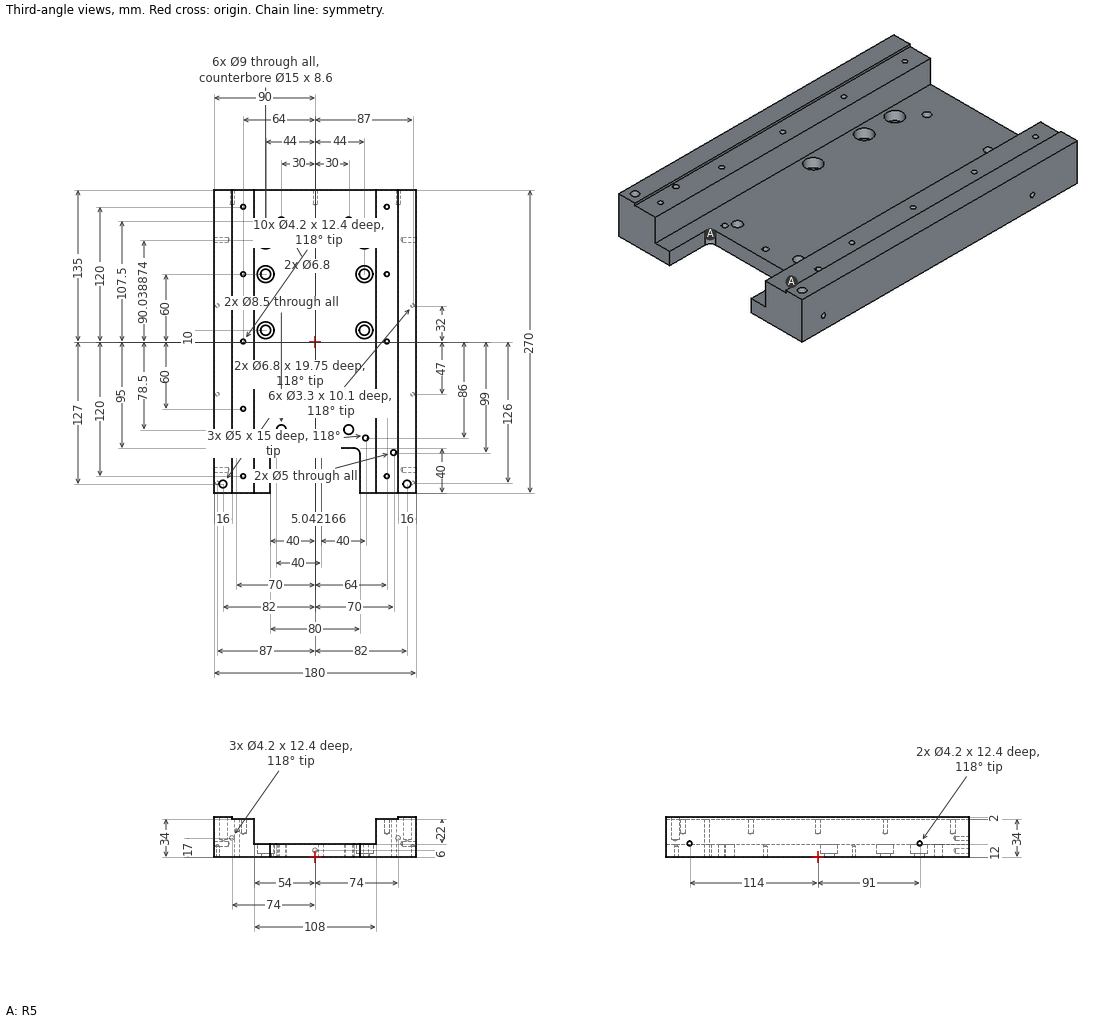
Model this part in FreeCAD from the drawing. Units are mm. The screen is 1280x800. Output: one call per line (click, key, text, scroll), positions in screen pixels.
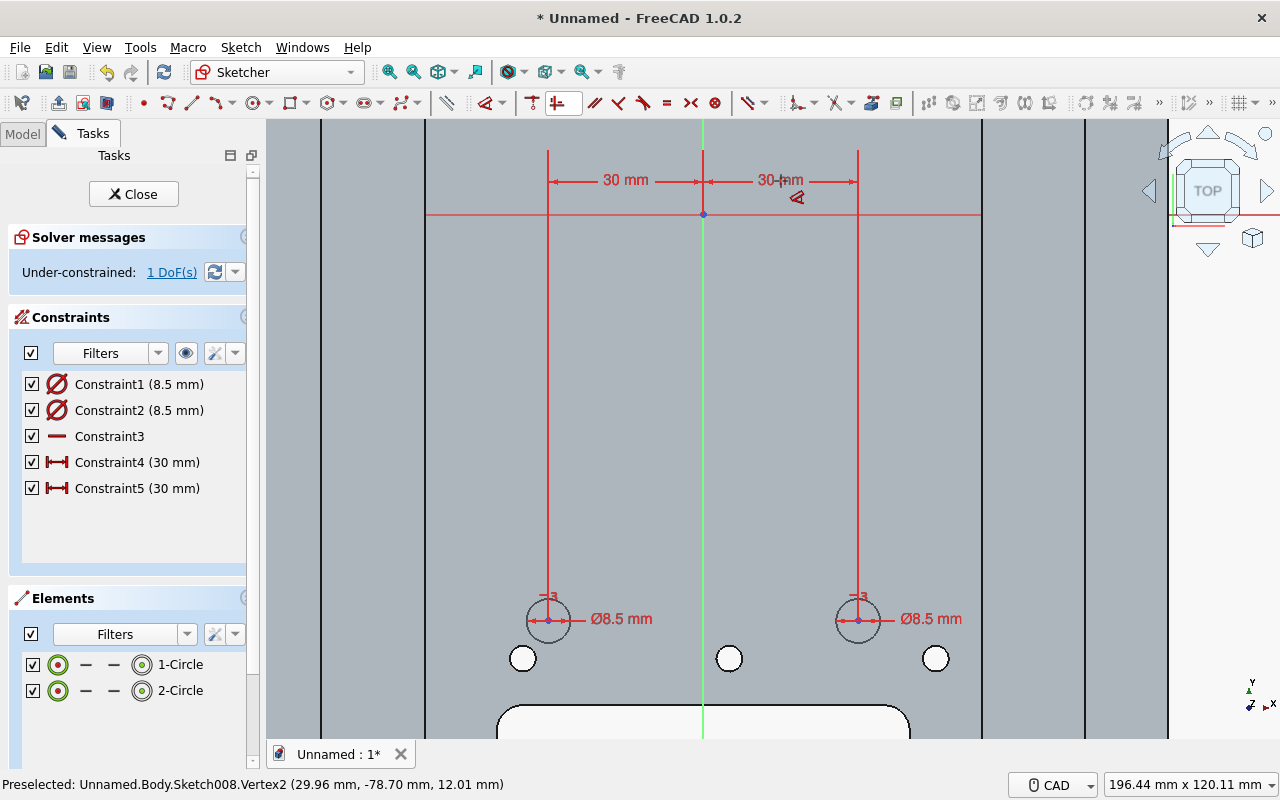
click(548, 621)
click(514, 418)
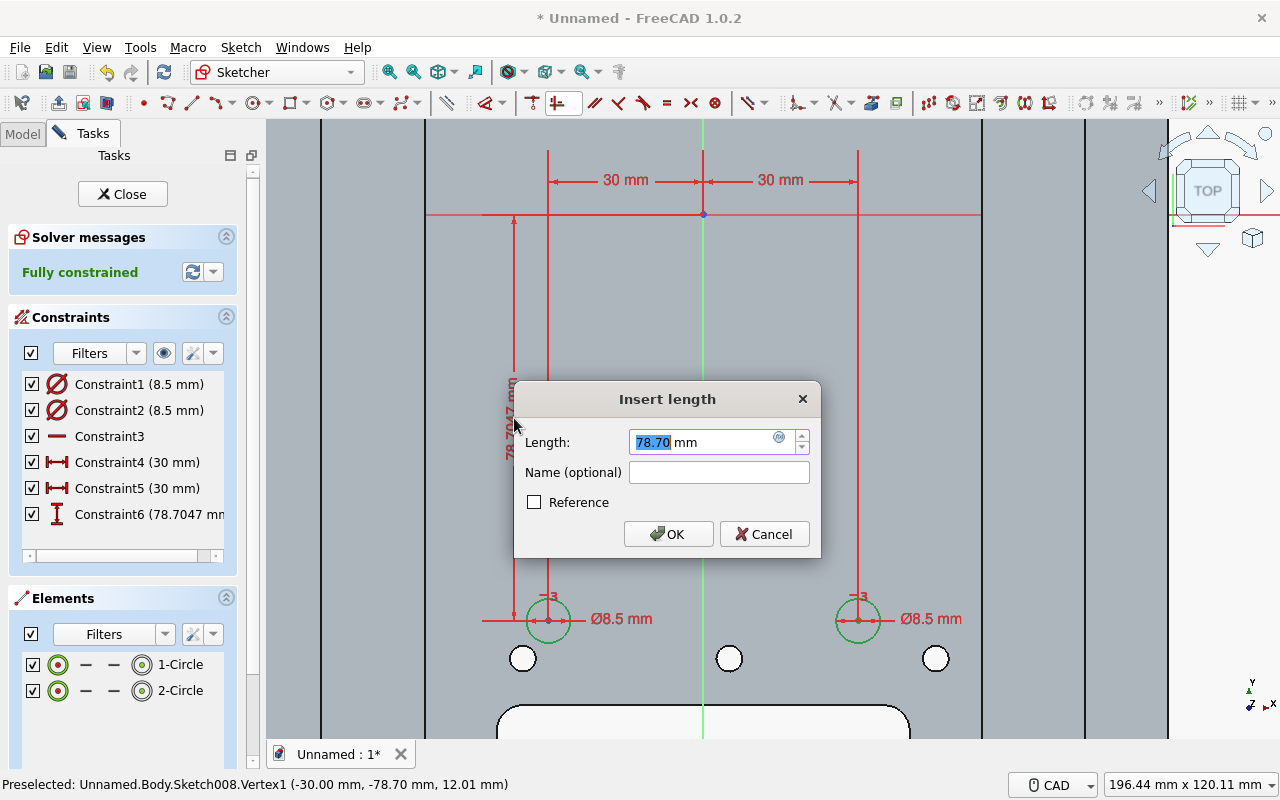
text(78.5)
key(Return)
key(Escape)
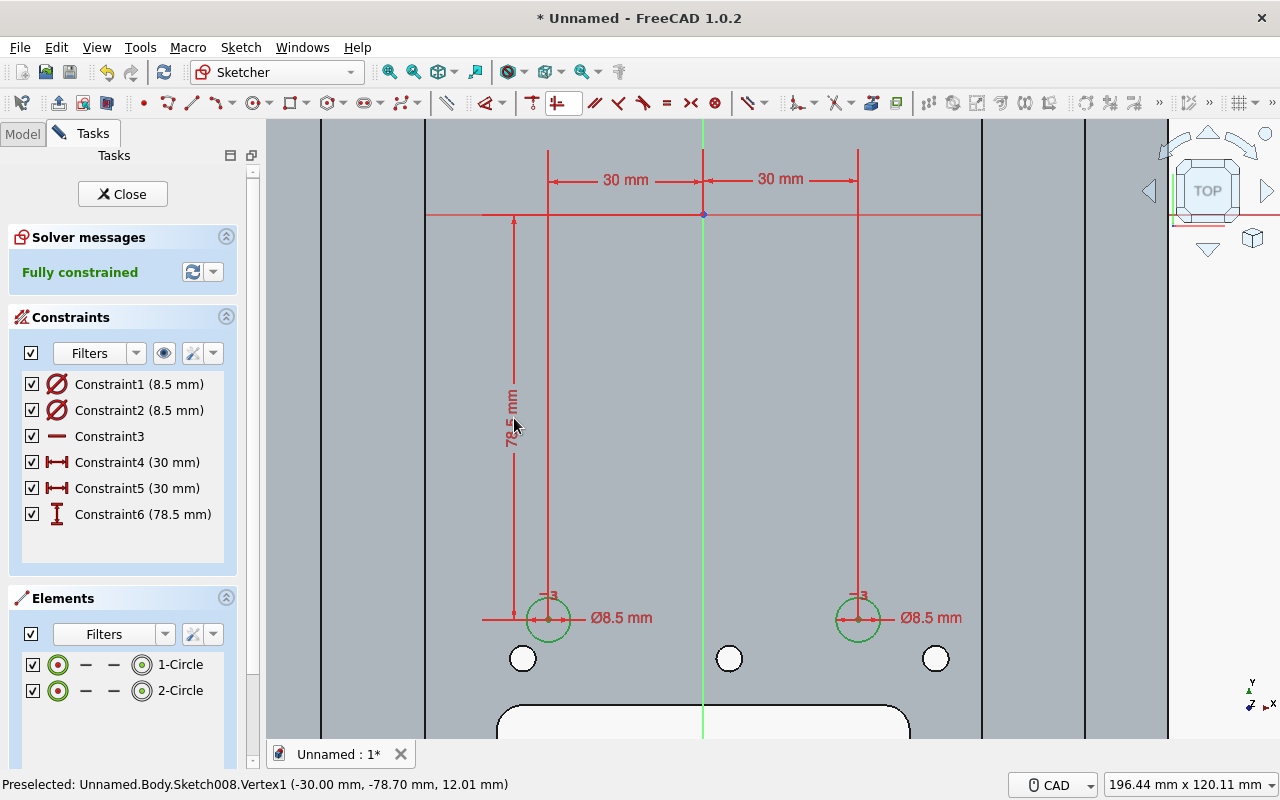
click(123, 194)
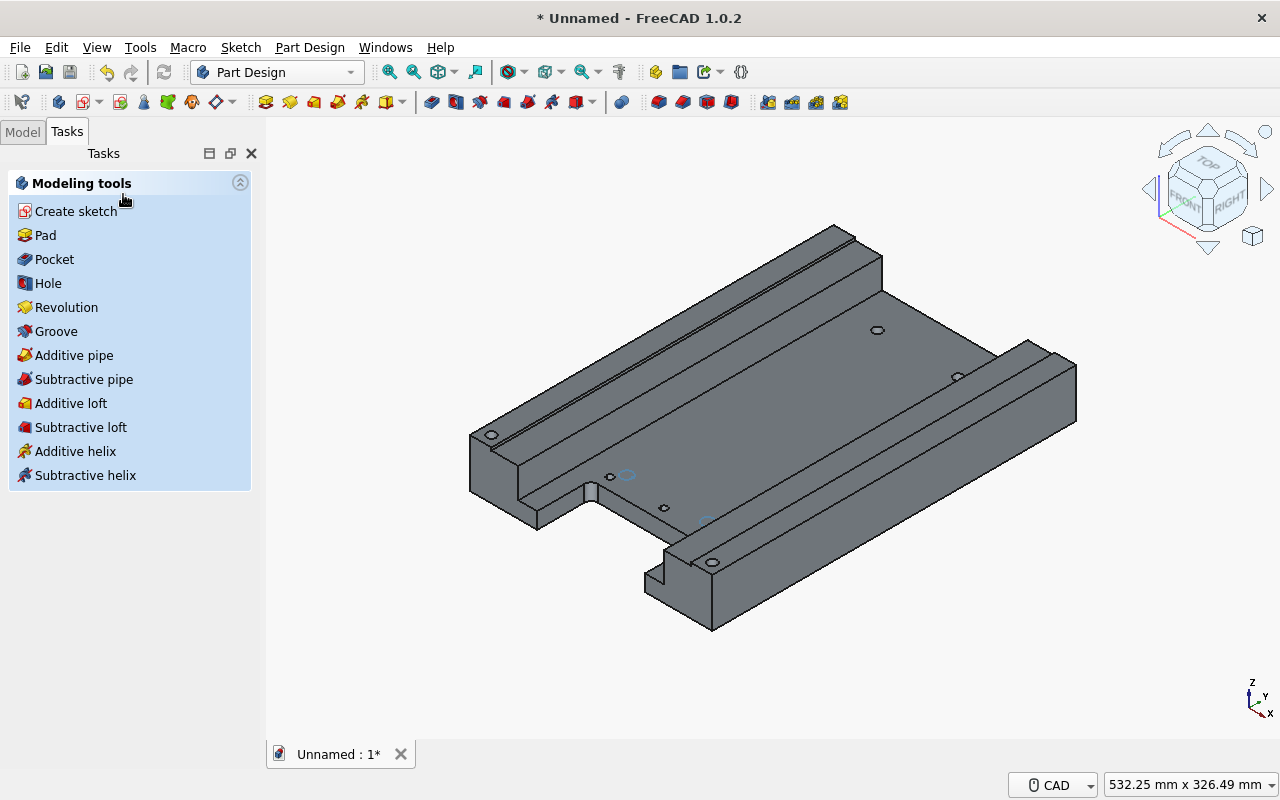
click(456, 102)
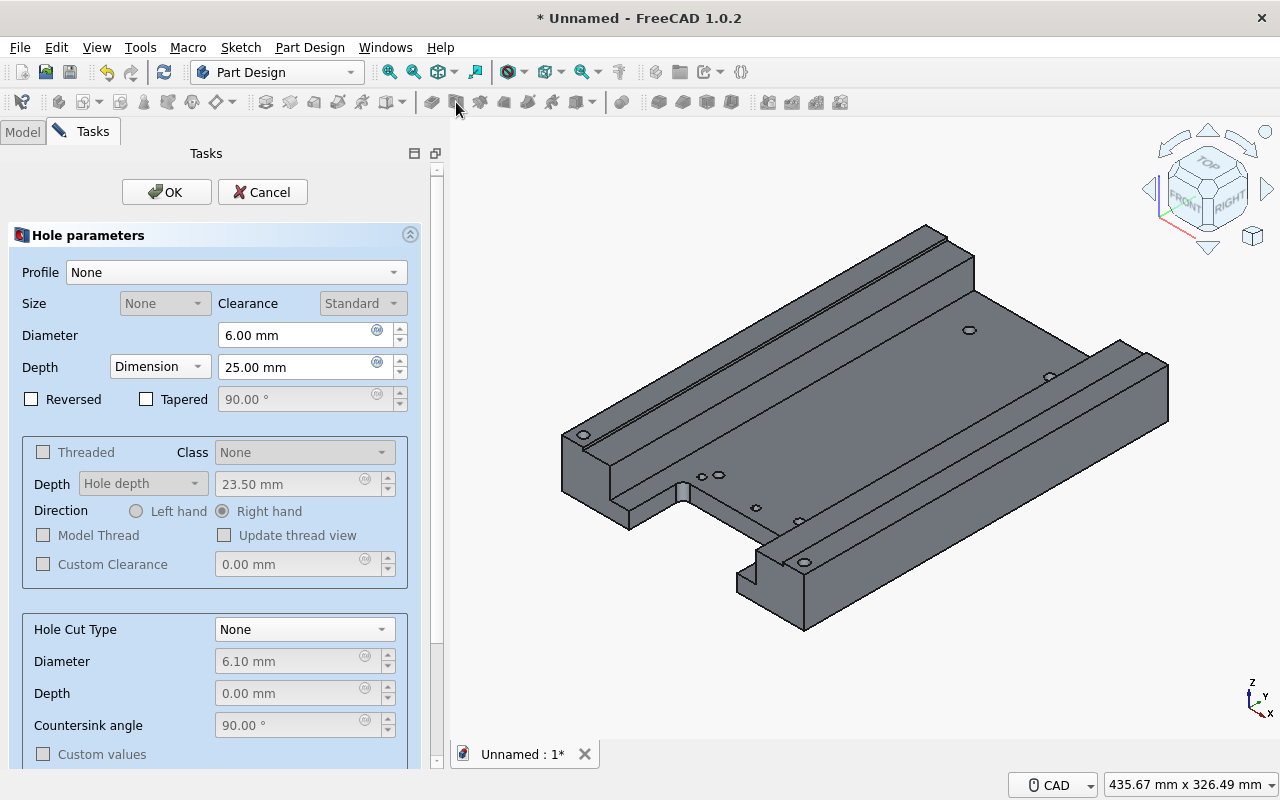
triple_click(305, 335)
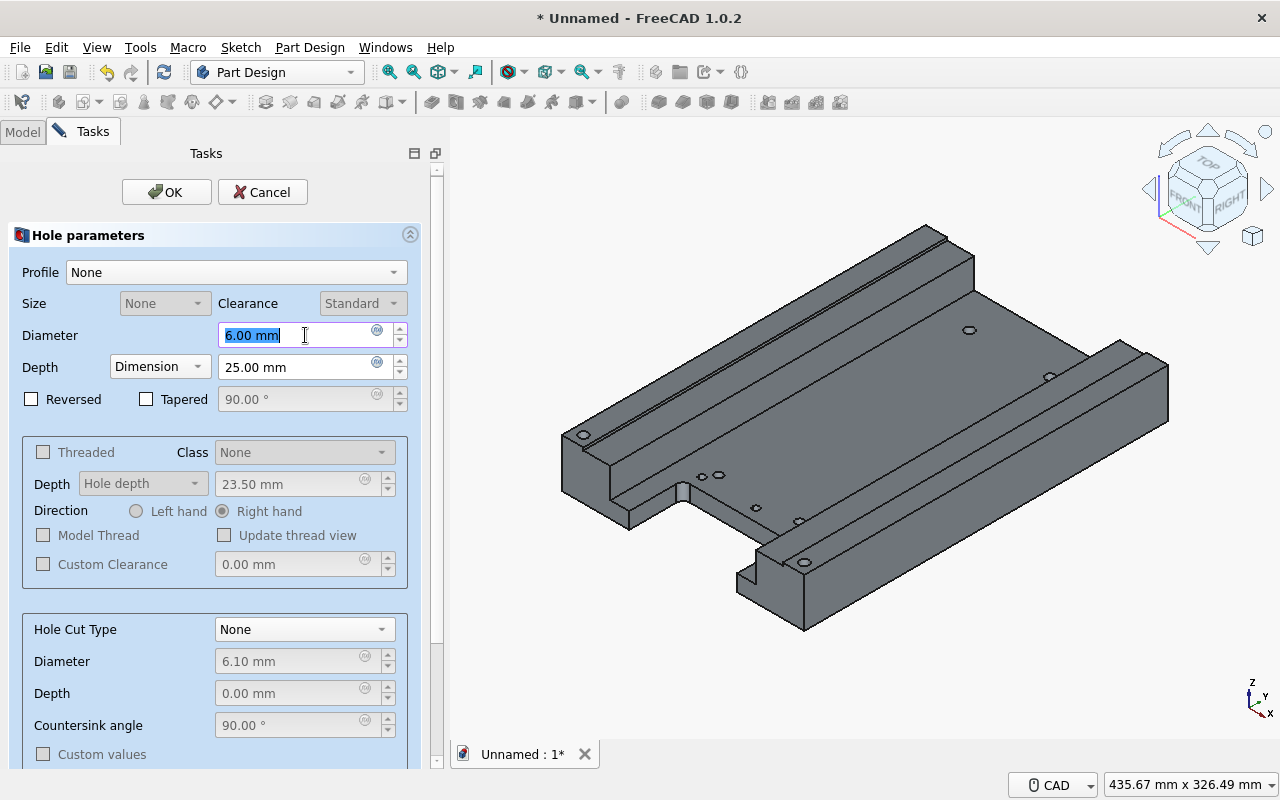
text(8.5)
key(Tab)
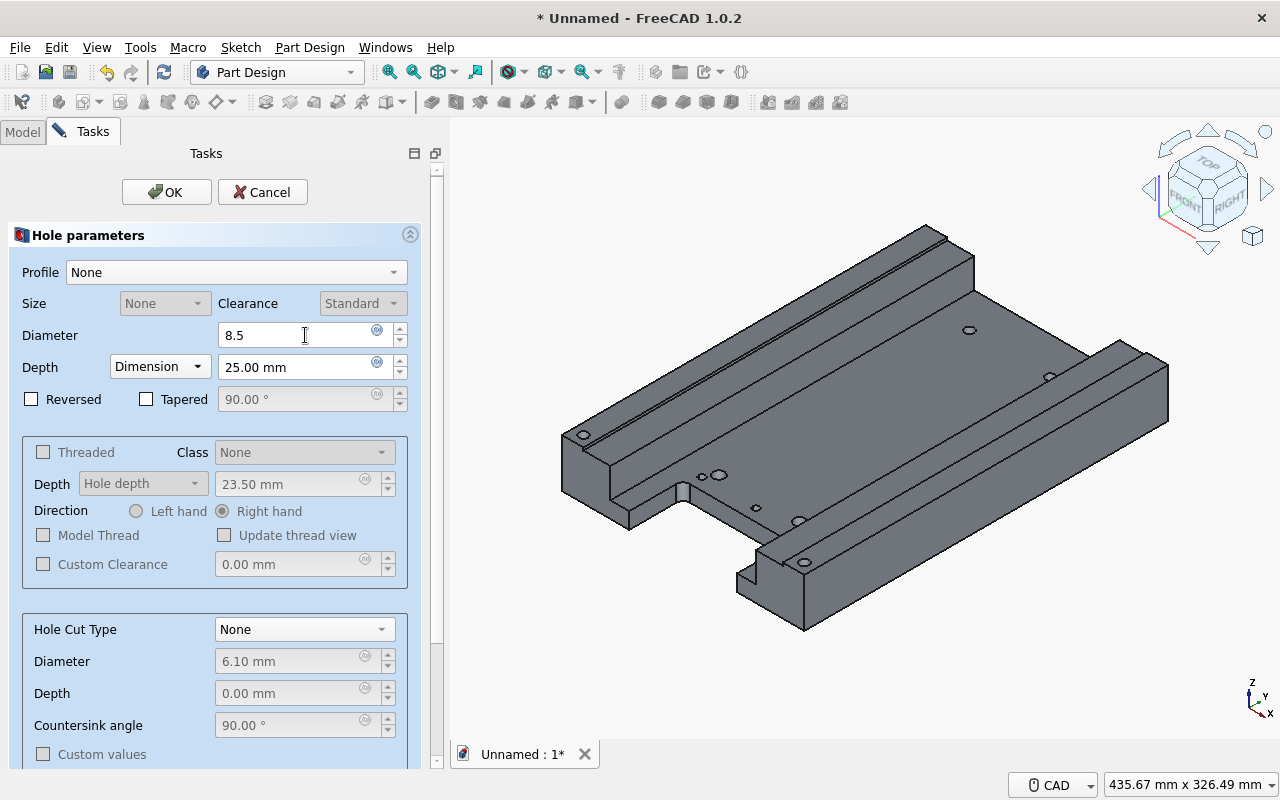
click(161, 366)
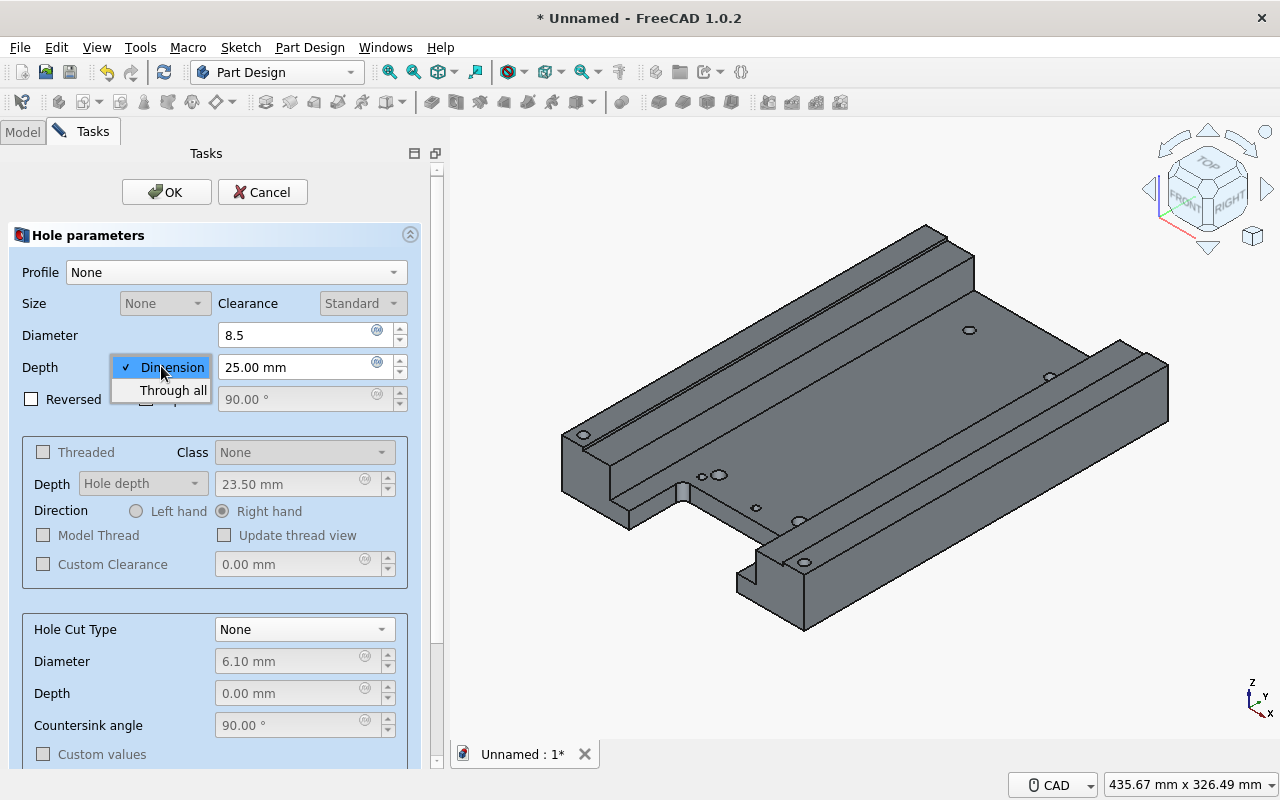
click(160, 390)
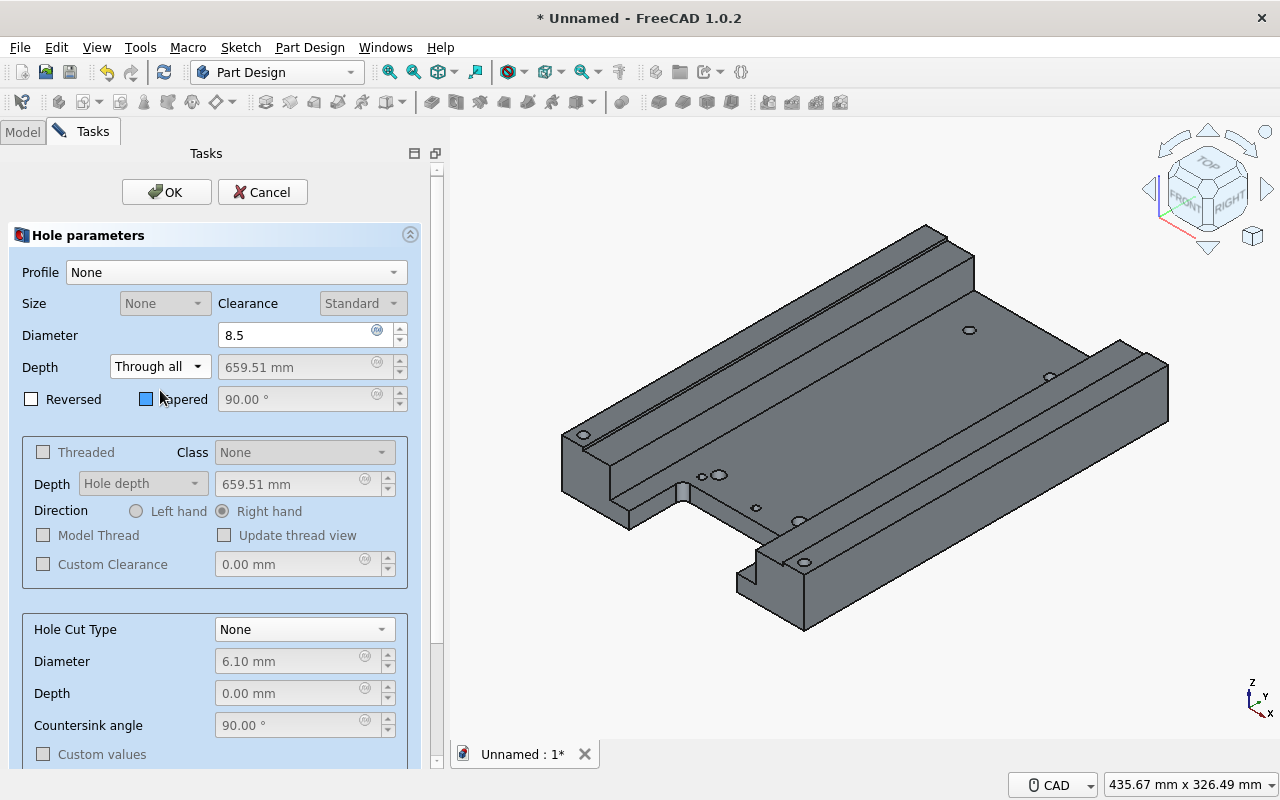
click(167, 192)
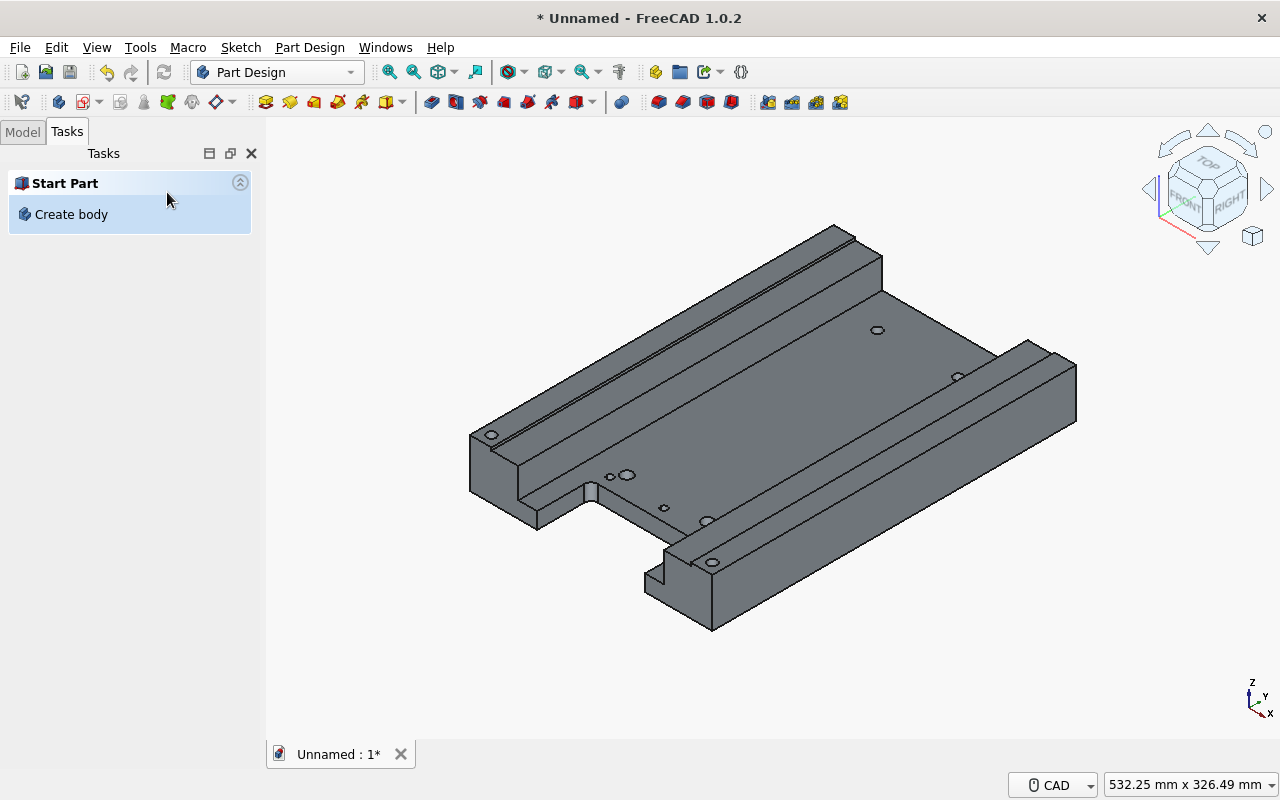
click(825, 406)